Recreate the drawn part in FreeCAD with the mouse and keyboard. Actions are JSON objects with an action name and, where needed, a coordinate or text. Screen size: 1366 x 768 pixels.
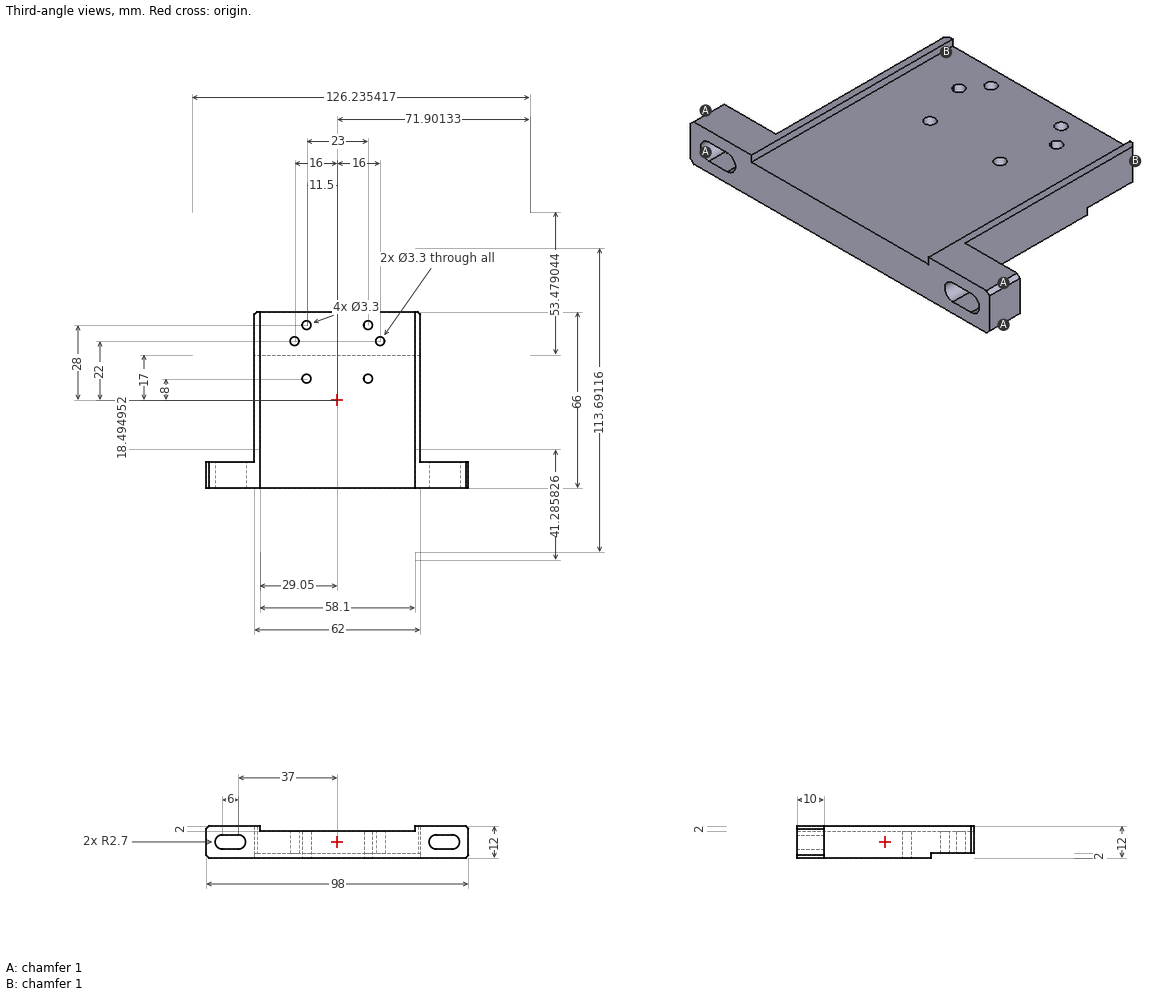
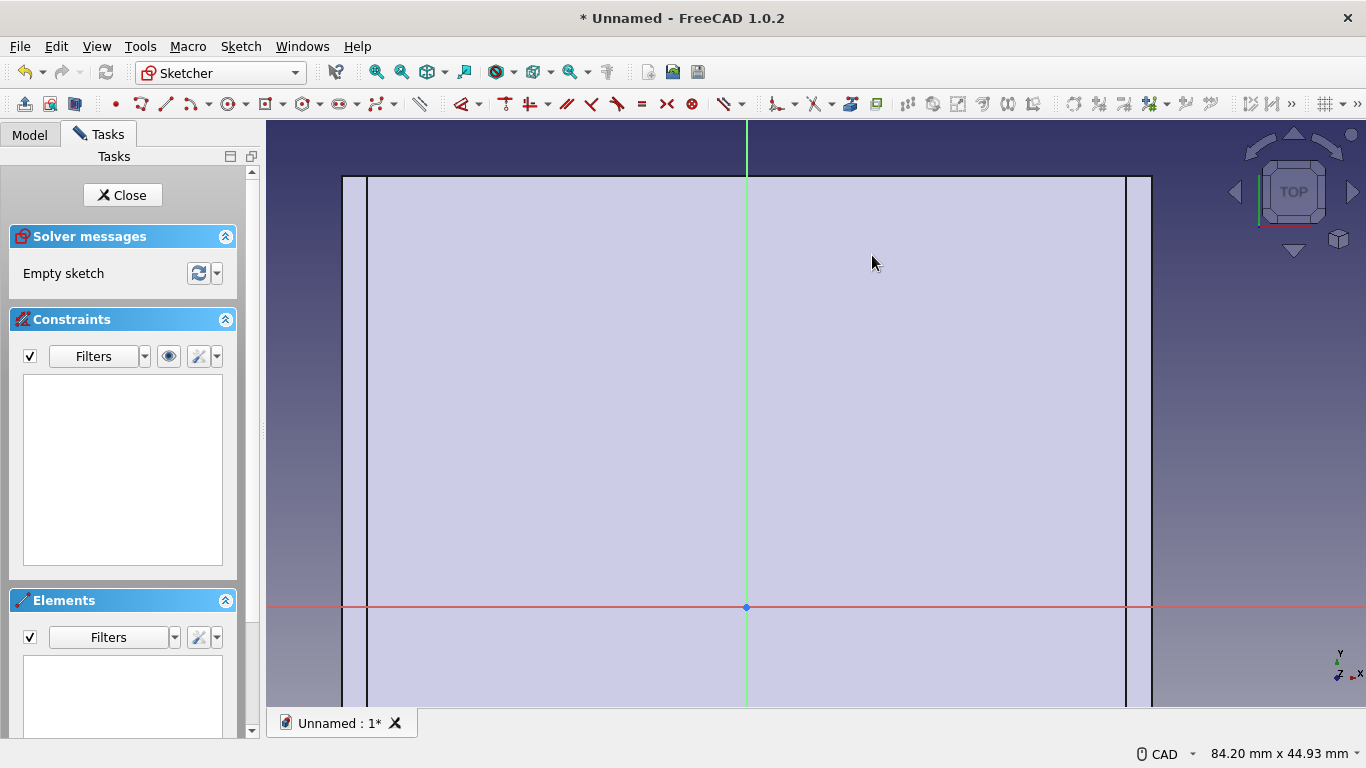
{"action": "left_click", "coordinate": [228, 104]}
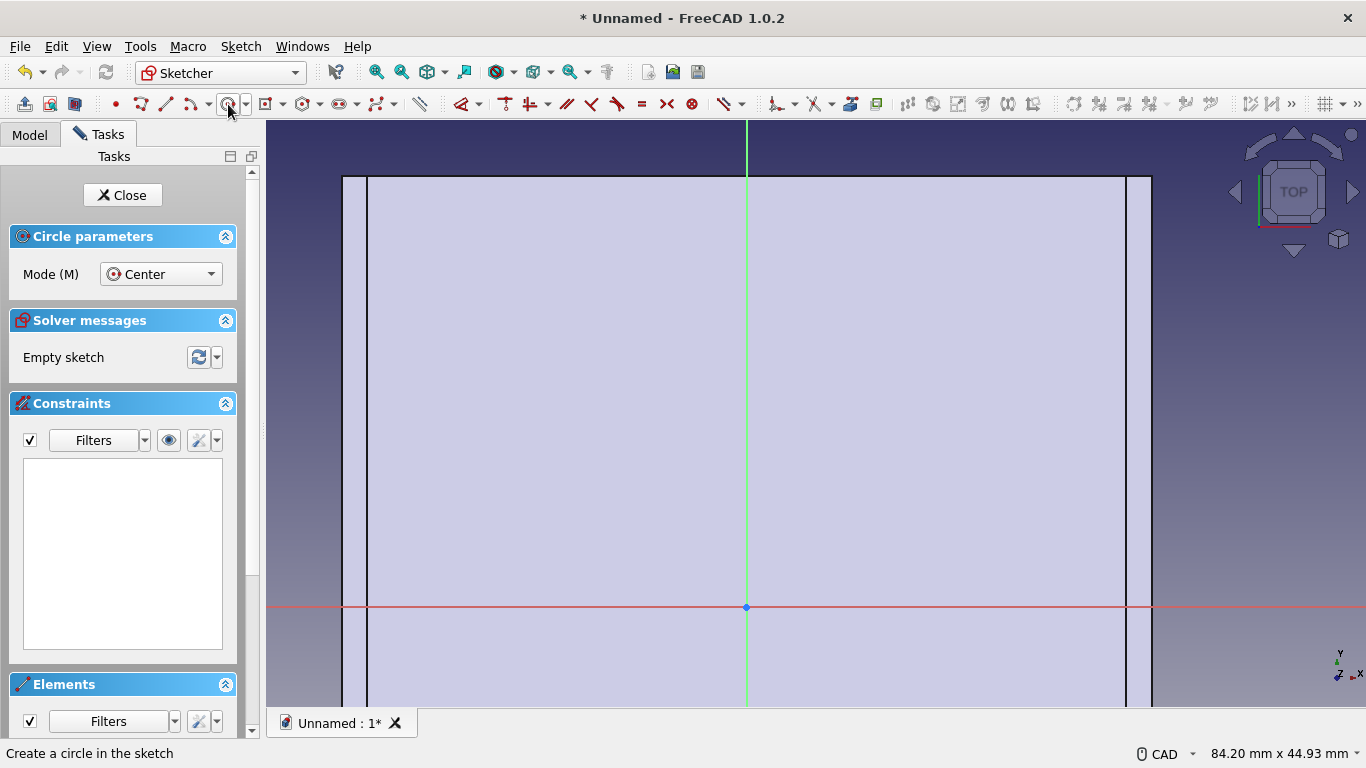
{"action": "left_click", "coordinate": [596, 242]}
{"action": "mouse_move", "coordinate": [612, 226]}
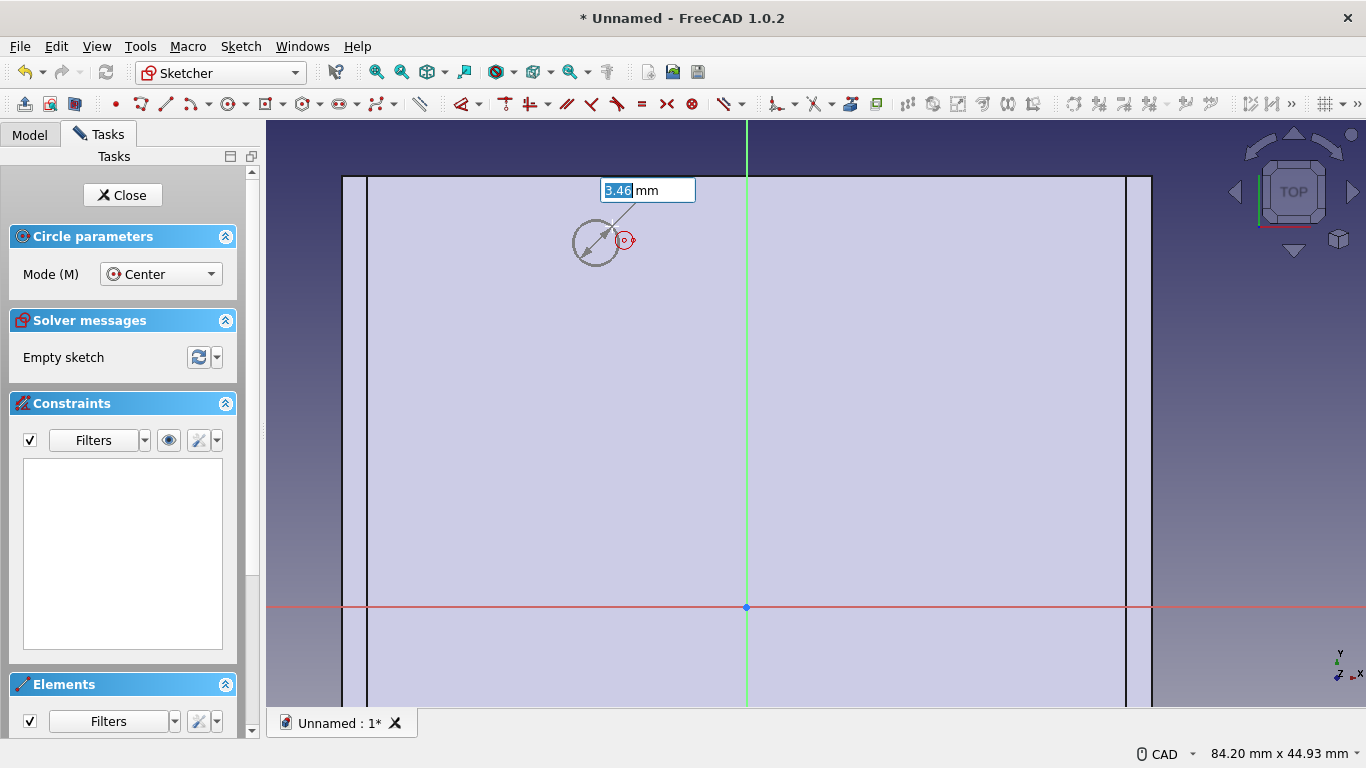
{"action": "type", "text": "3.3"}
{"action": "key", "text": "Return"}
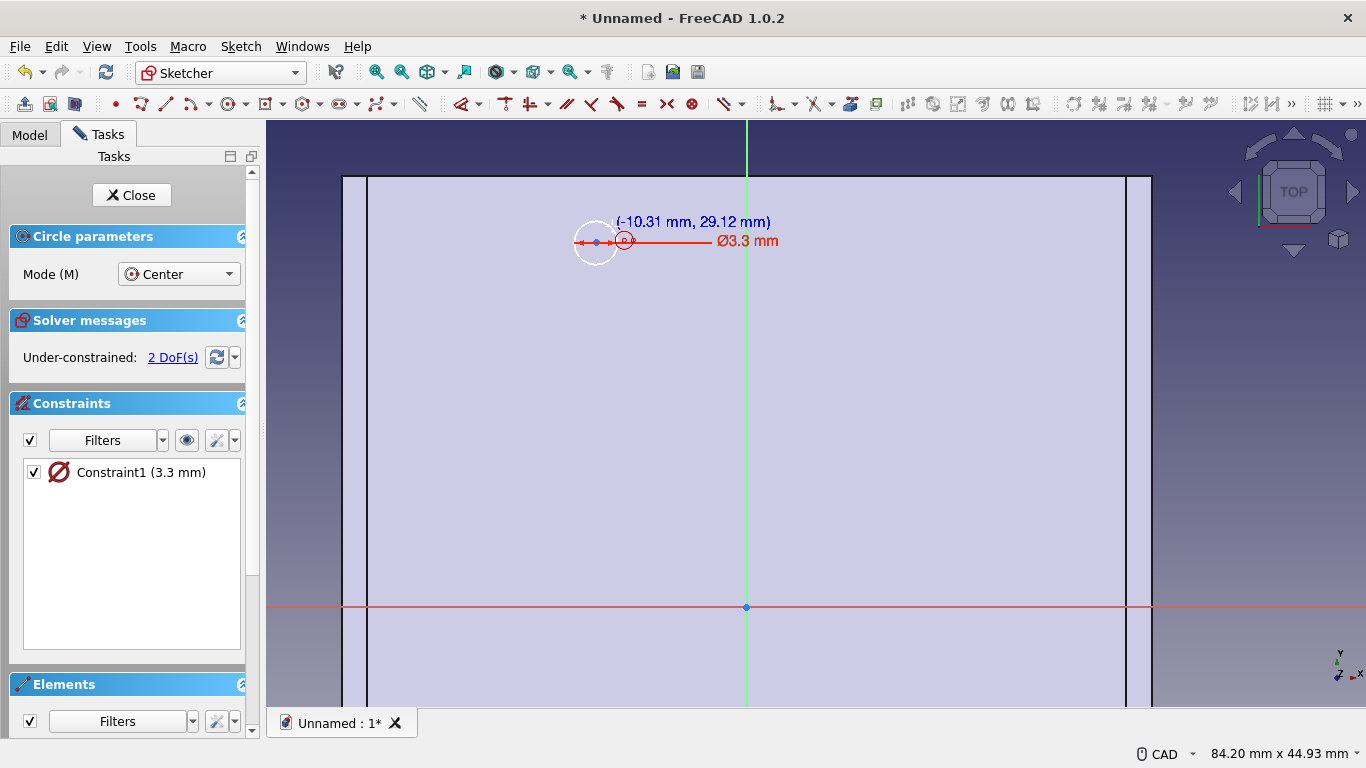
{"action": "left_click", "coordinate": [897, 242]}
{"action": "mouse_move", "coordinate": [912, 226]}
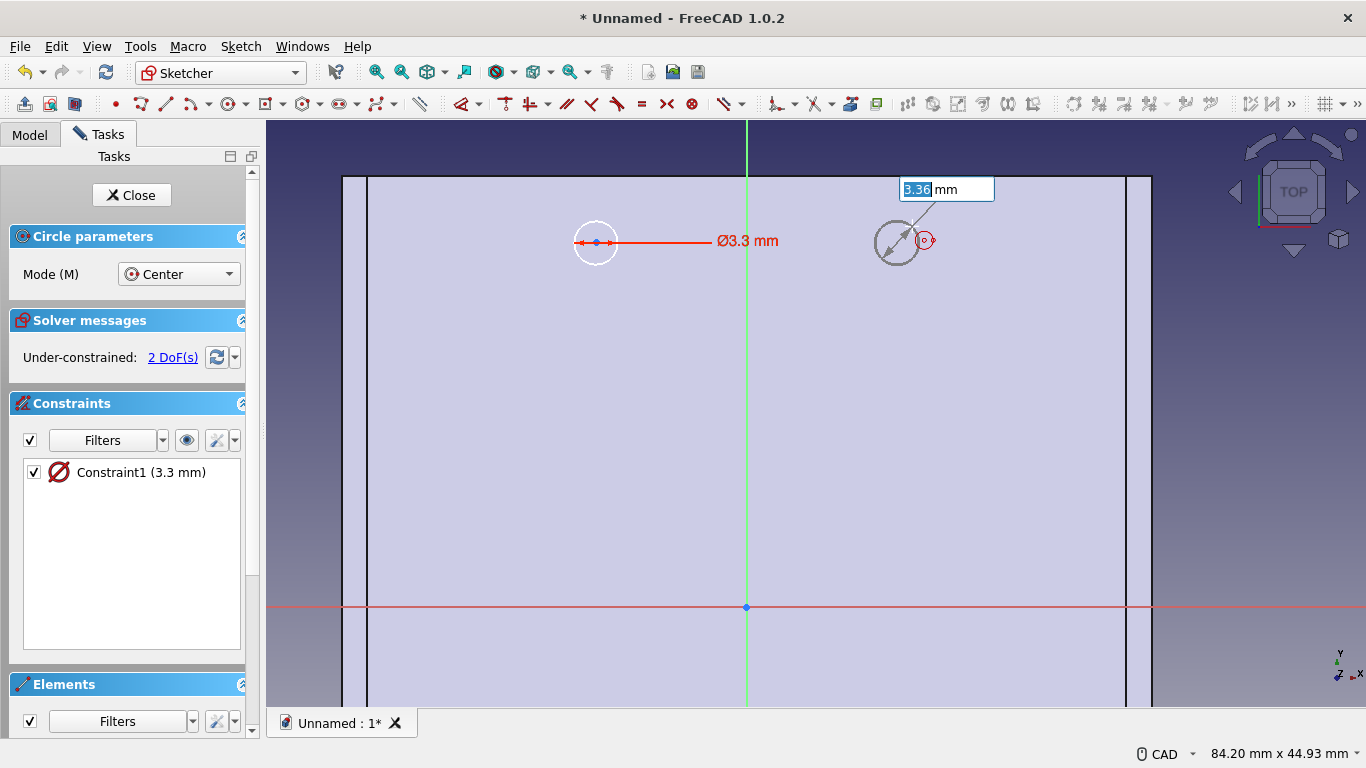
{"action": "type", "text": "3.3"}
{"action": "key", "text": "Return"}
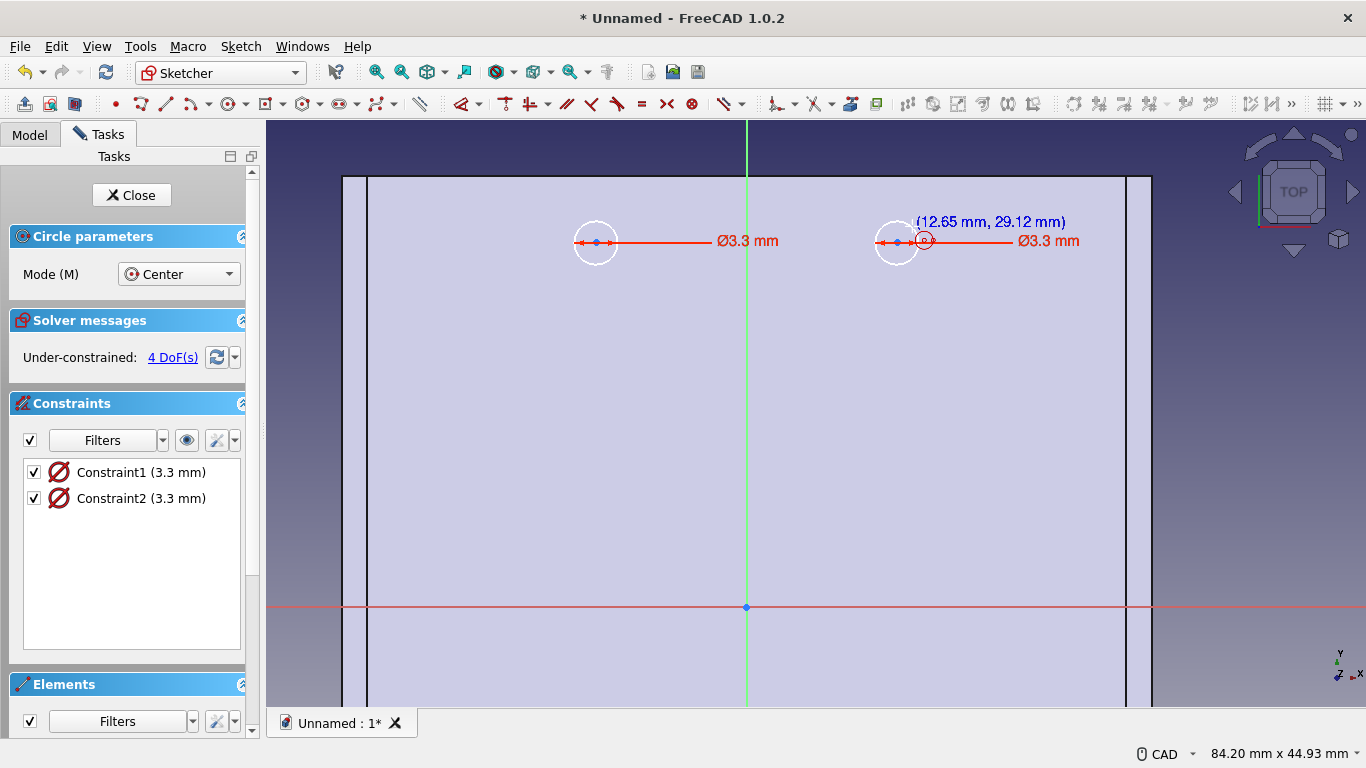
{"action": "left_click", "coordinate": [596, 503]}
{"action": "mouse_move", "coordinate": [612, 488]}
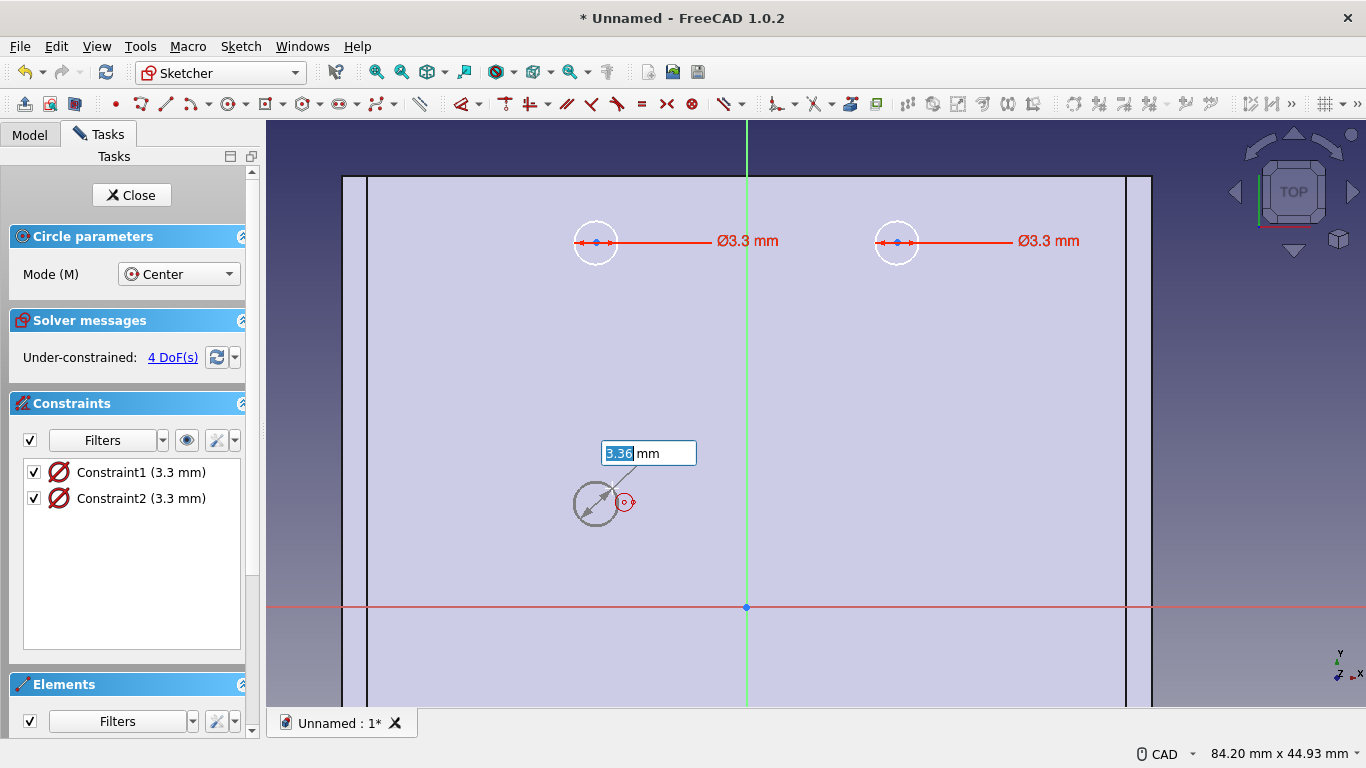
{"action": "type", "text": "3.3"}
{"action": "key", "text": "Return"}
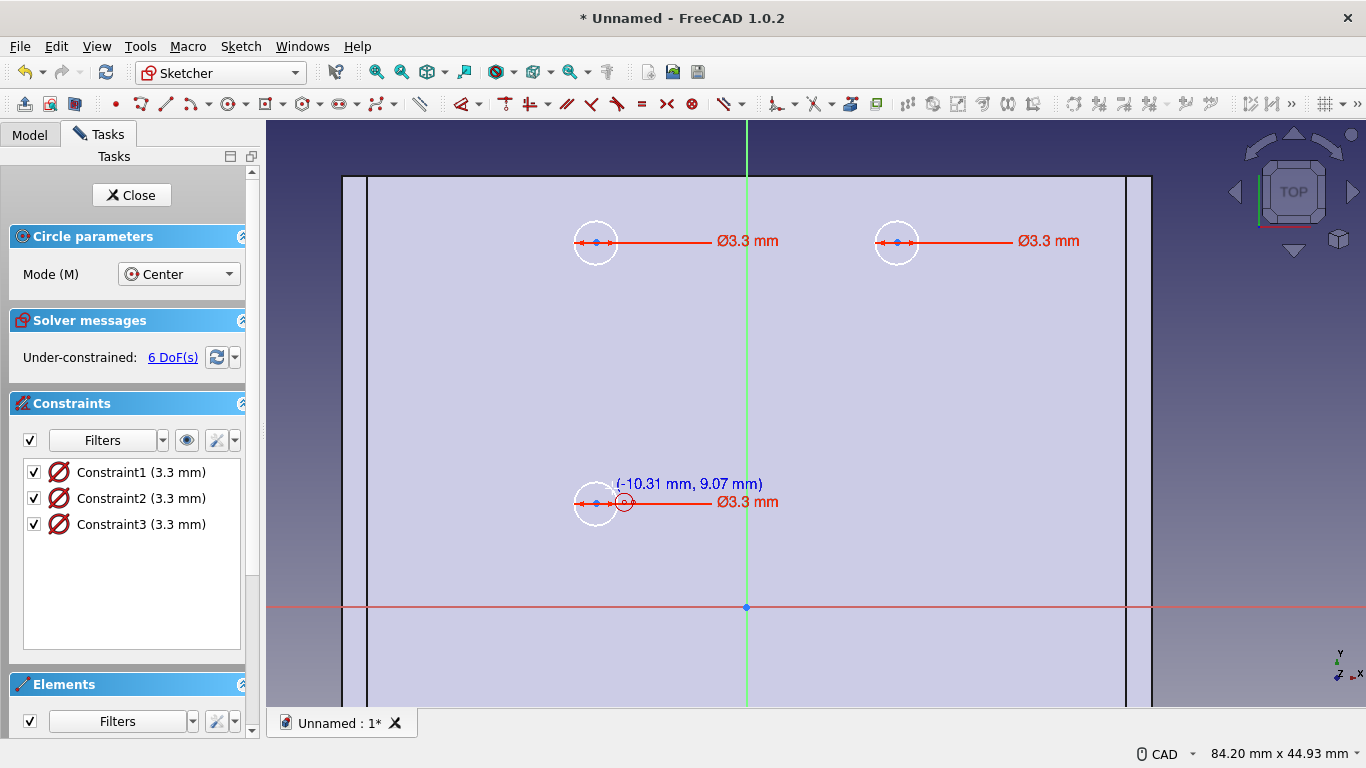
{"action": "left_click", "coordinate": [897, 503]}
{"action": "mouse_move", "coordinate": [912, 488]}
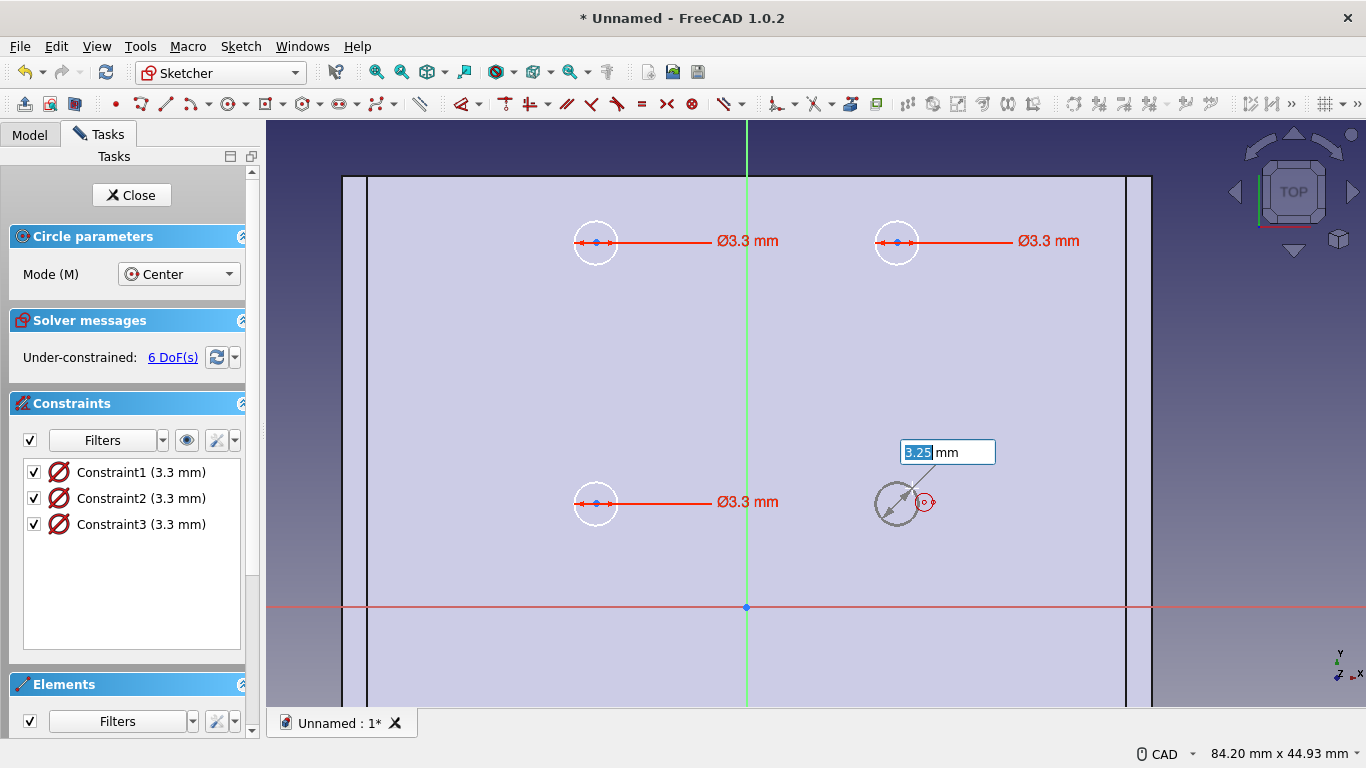
{"action": "type", "text": "3.3"}
{"action": "key", "text": "Return"}
{"action": "key", "text": "Escape"}